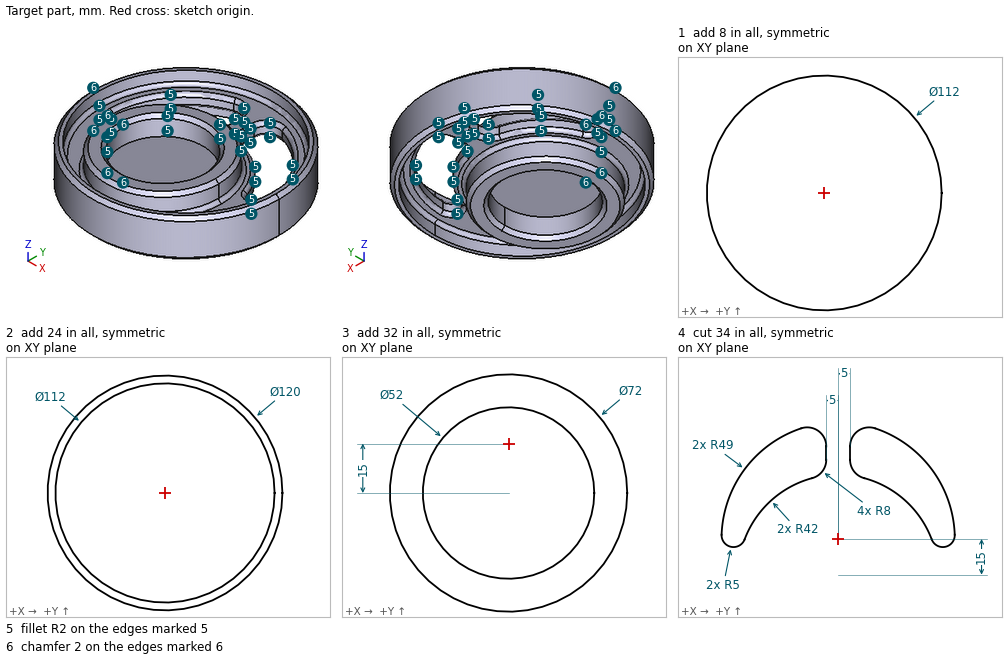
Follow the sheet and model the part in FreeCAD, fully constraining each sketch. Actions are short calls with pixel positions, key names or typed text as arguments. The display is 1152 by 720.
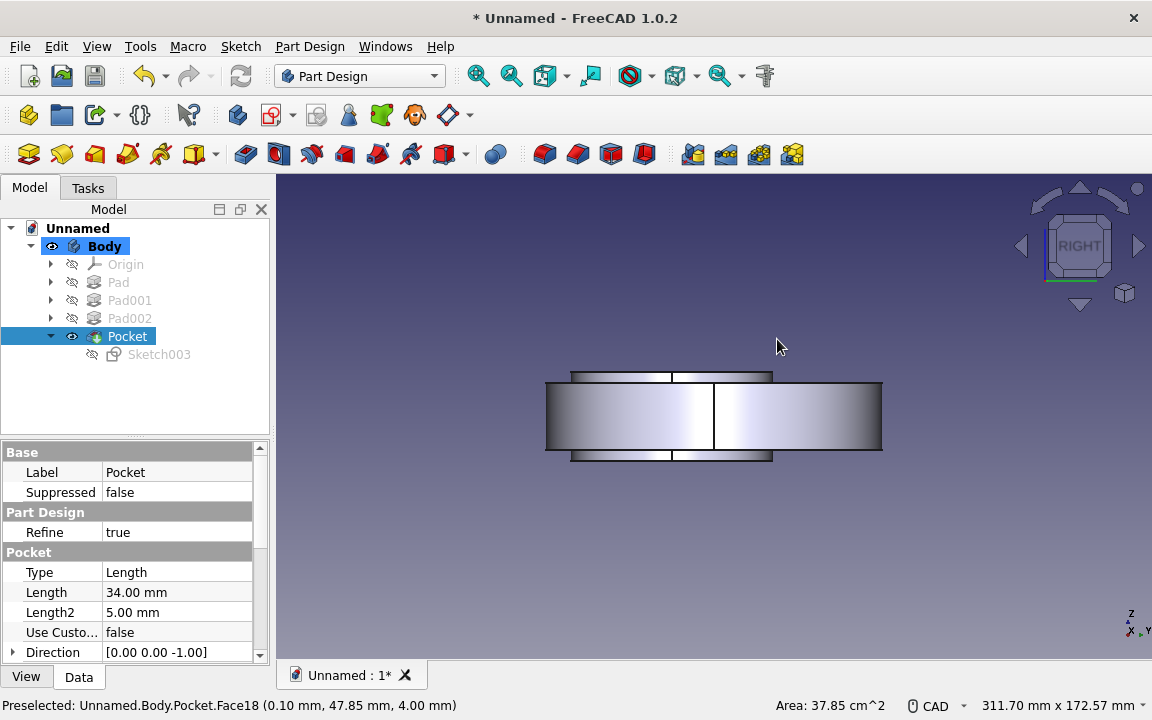
key(5)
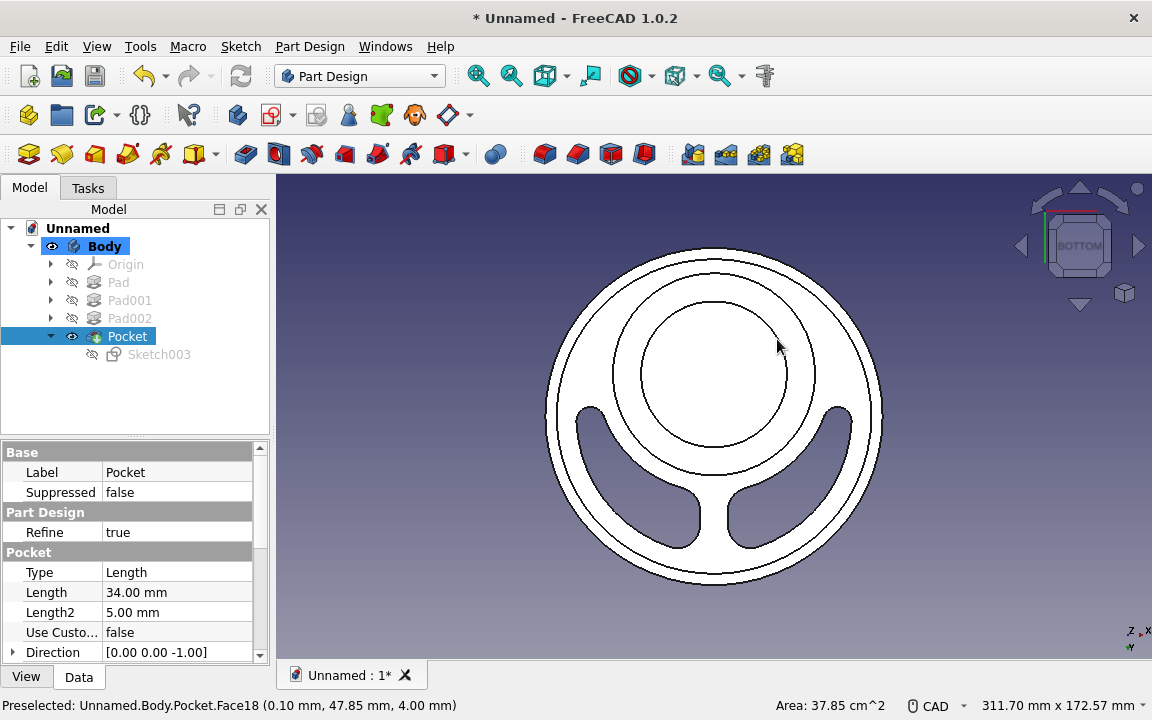
click(714, 550, ctrl)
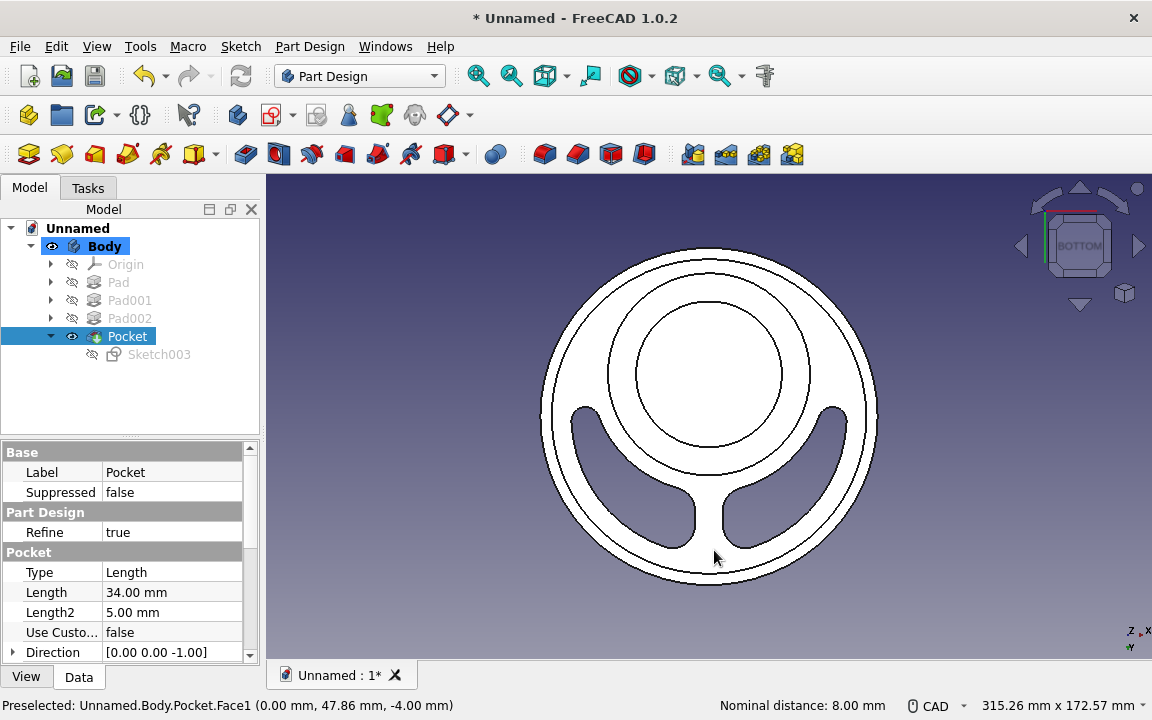
click(545, 154)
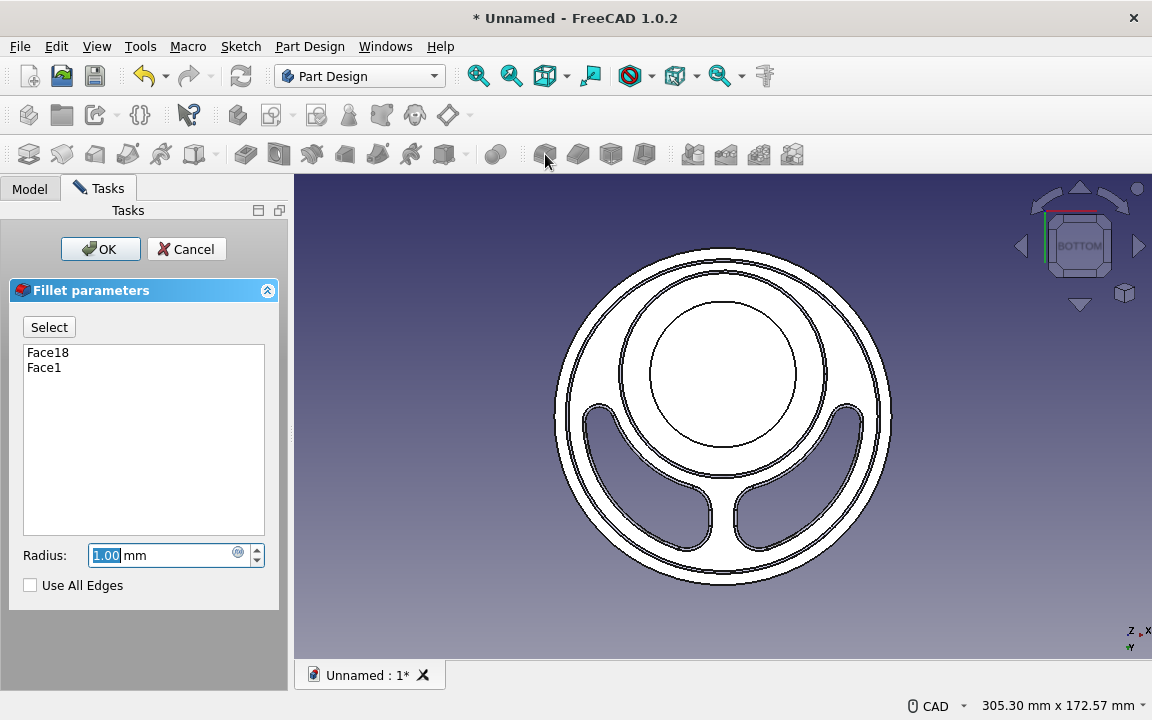
text(2)
key(Tab)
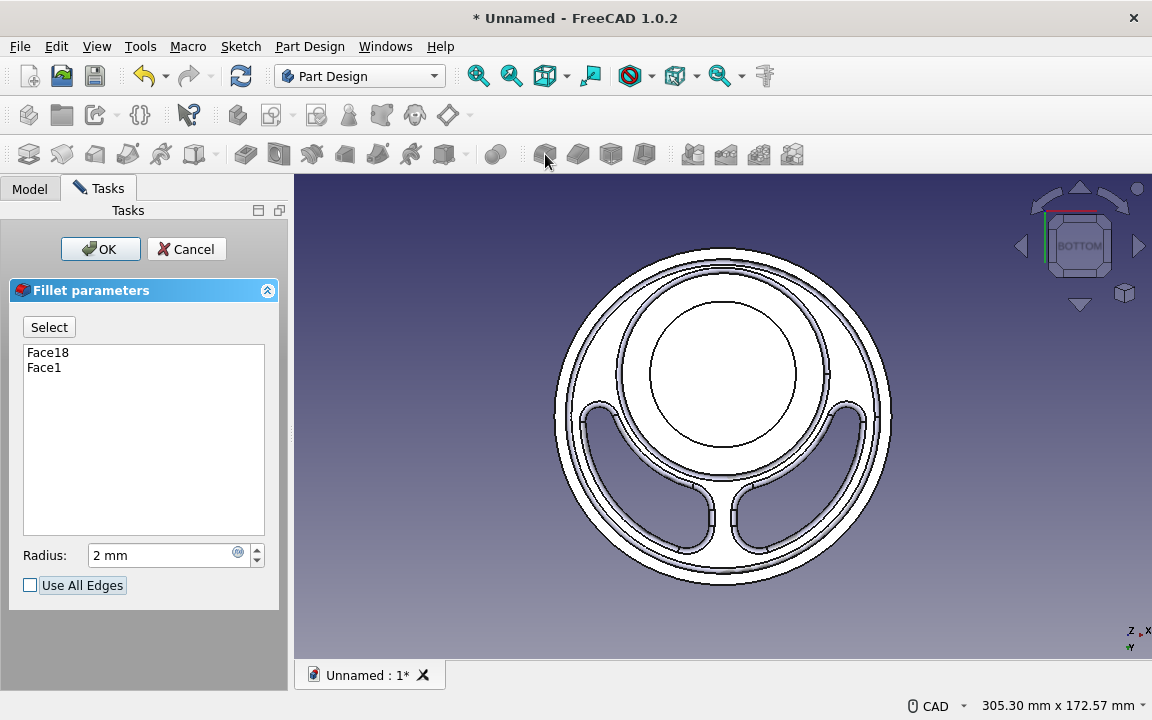
click(101, 249)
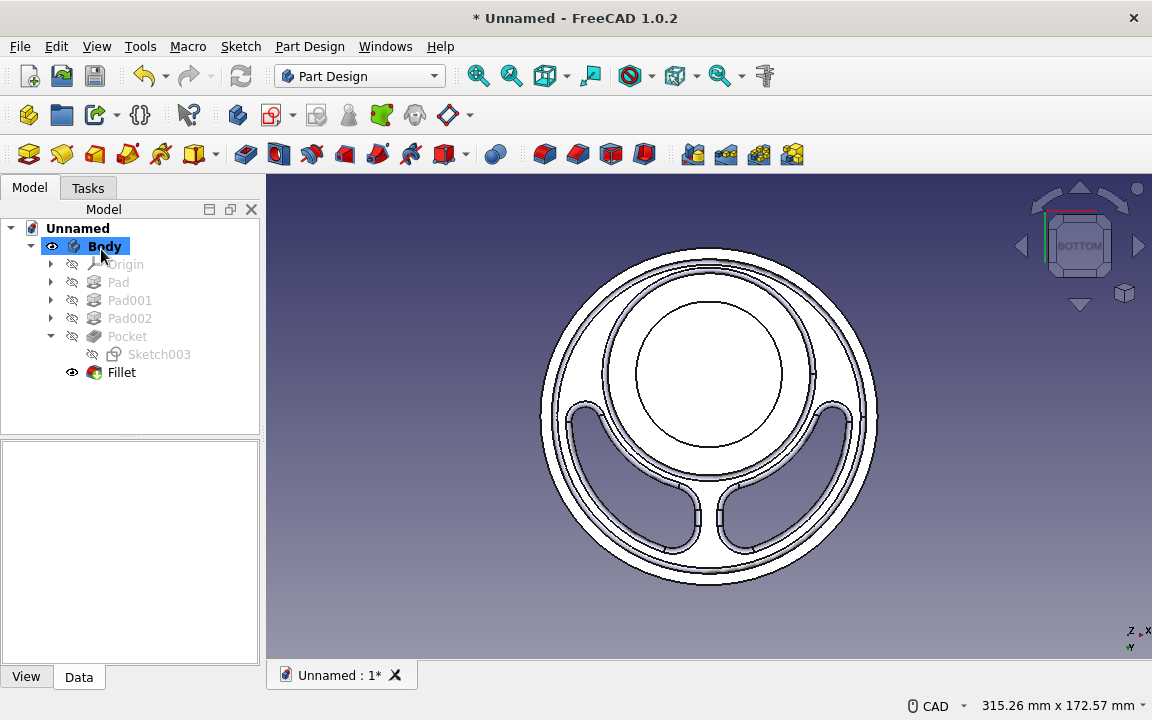
click(608, 373)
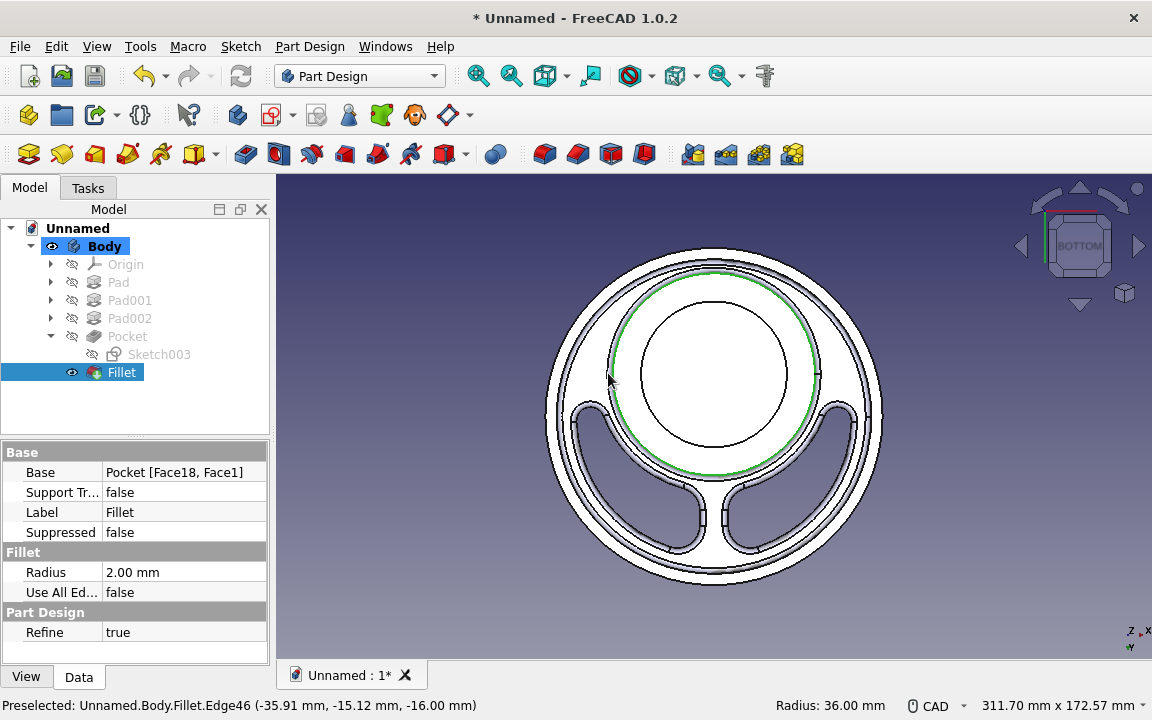
click(641, 373, ctrl)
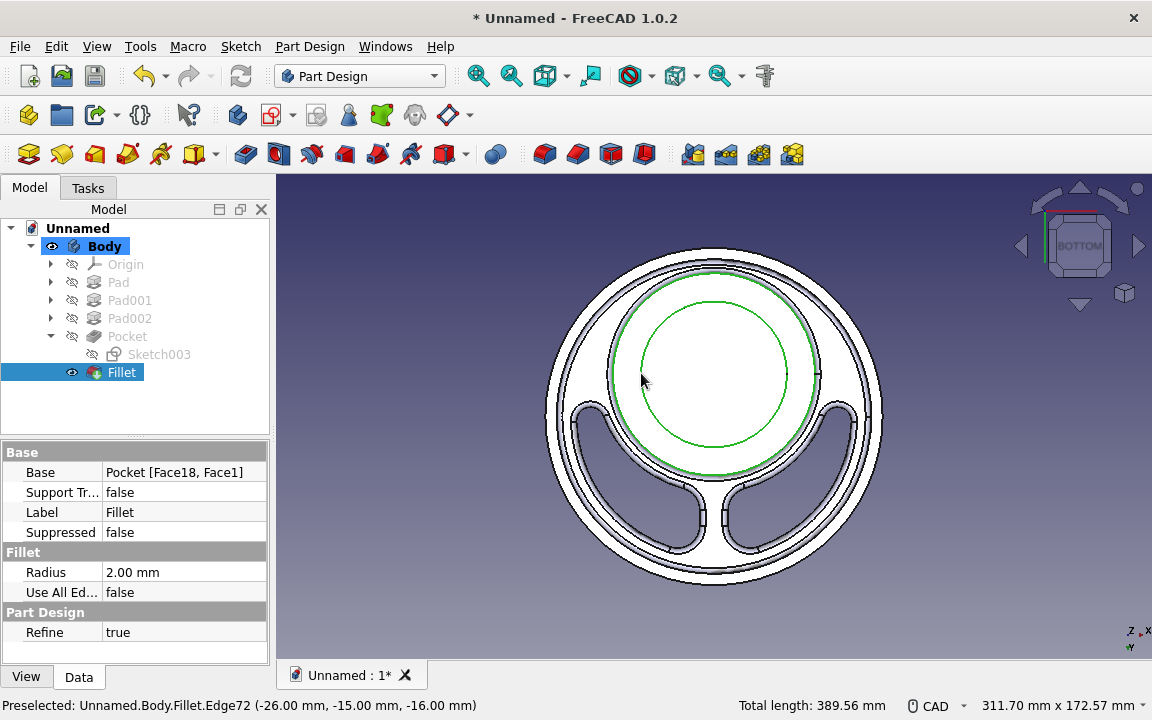
click(545, 415, ctrl)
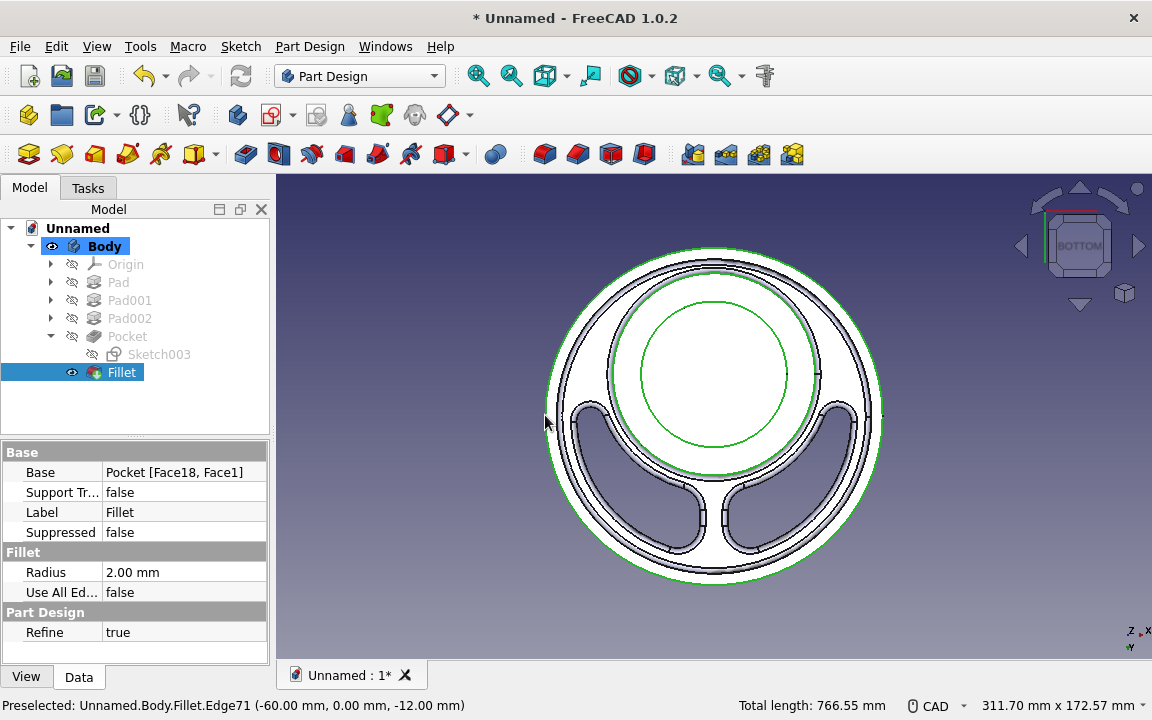
key(0)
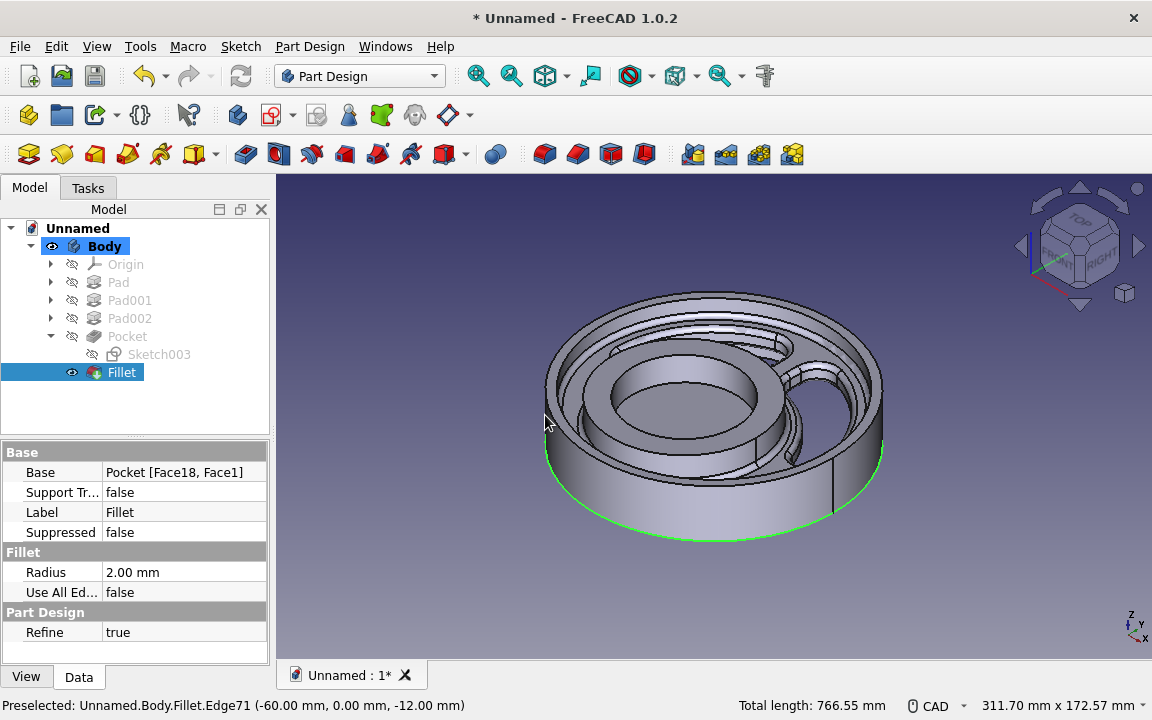
click(633, 366, ctrl)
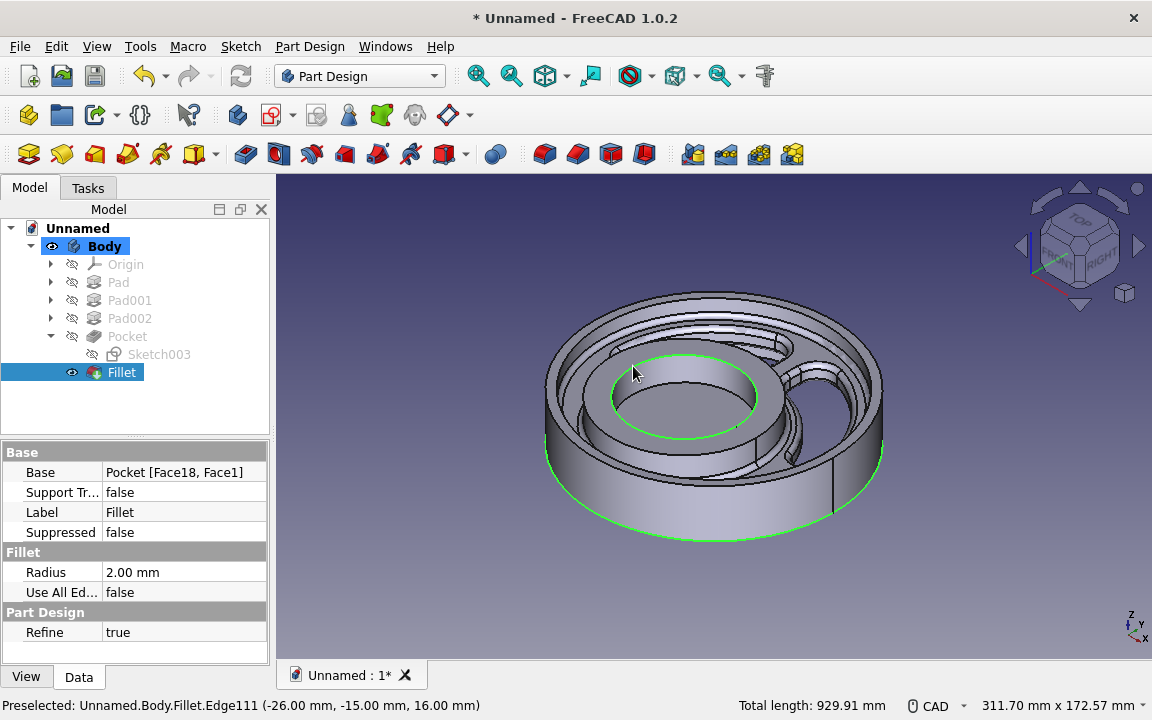
click(594, 423, ctrl)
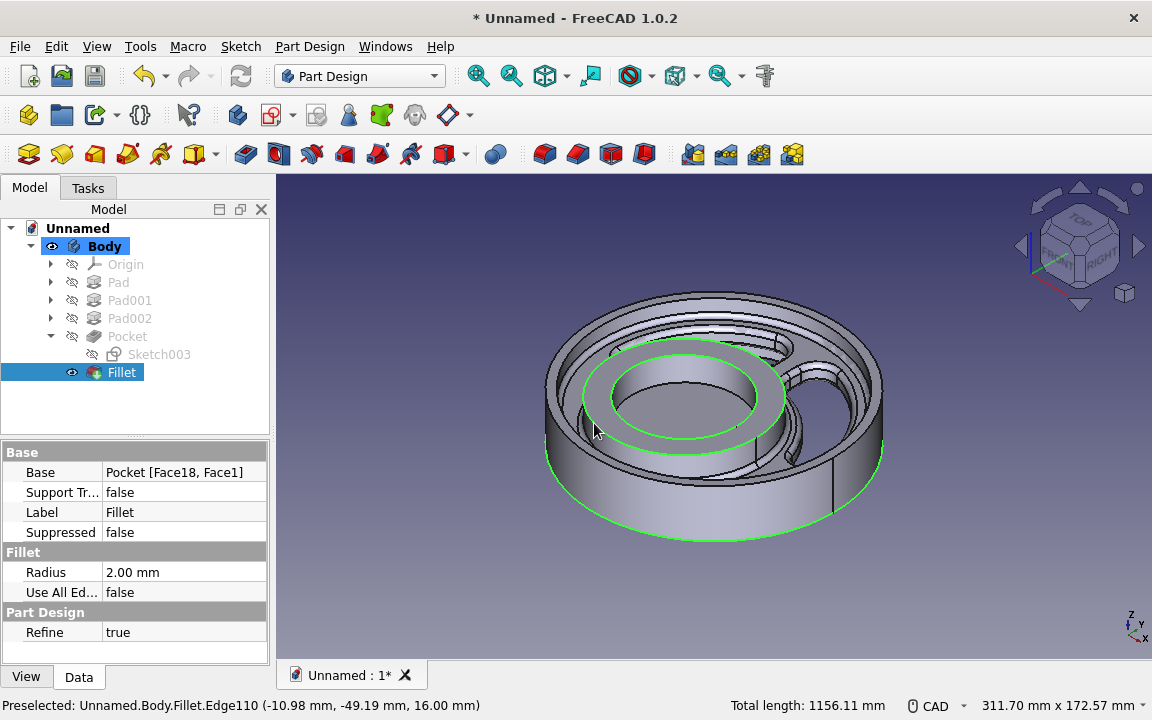
click(564, 432, ctrl)